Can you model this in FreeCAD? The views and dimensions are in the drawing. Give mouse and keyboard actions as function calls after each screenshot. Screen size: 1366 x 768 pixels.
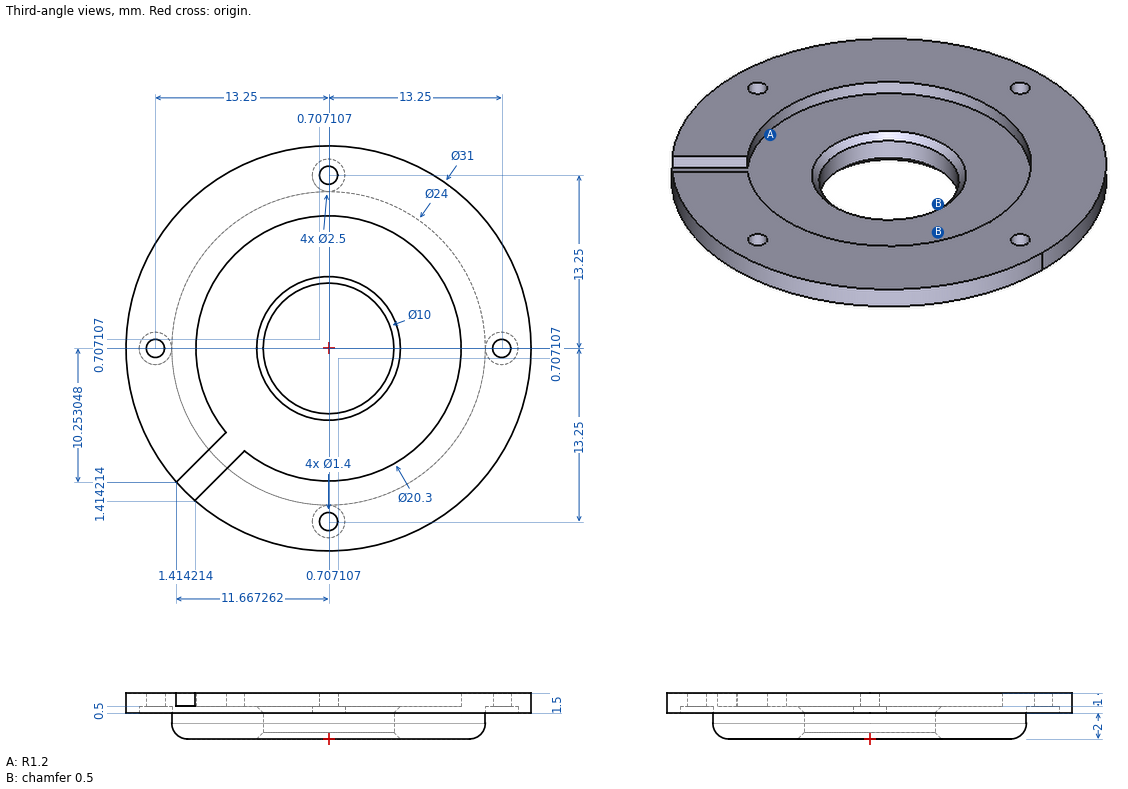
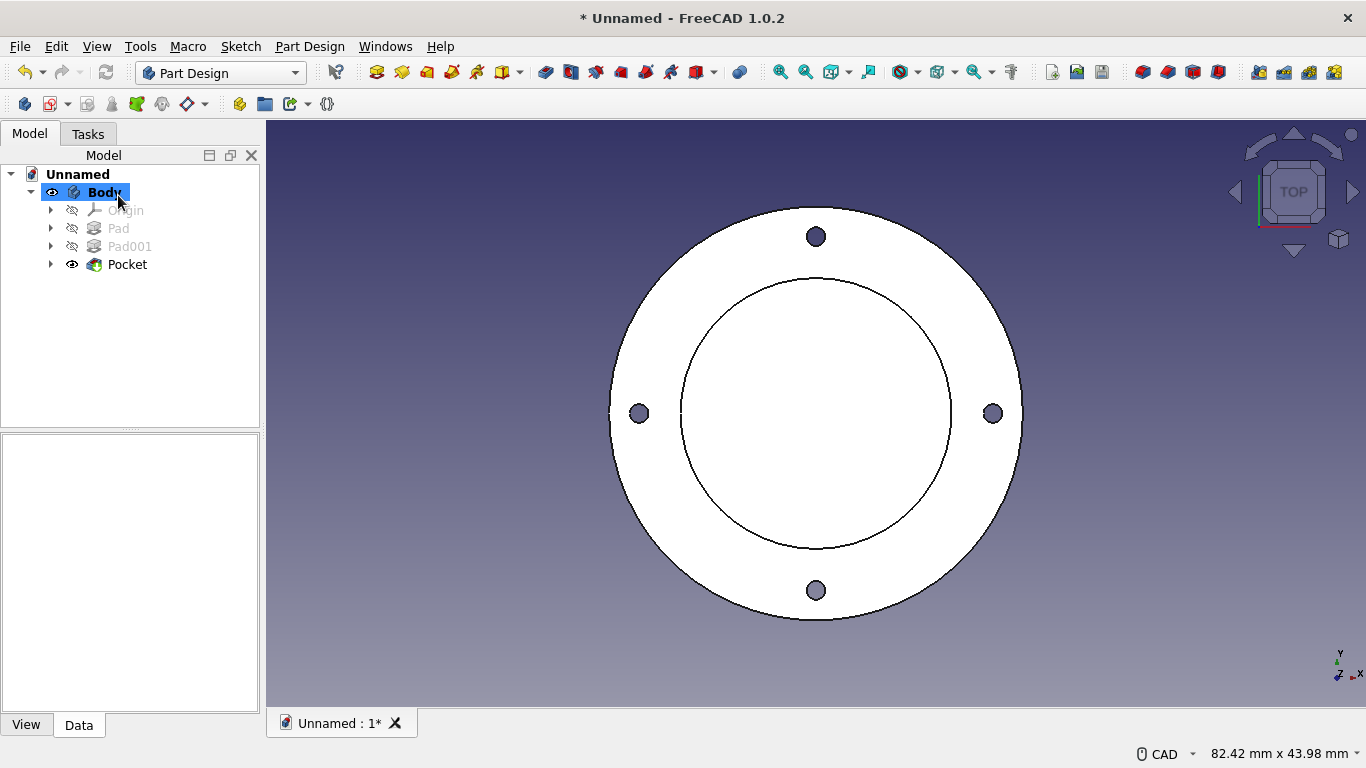
key(1)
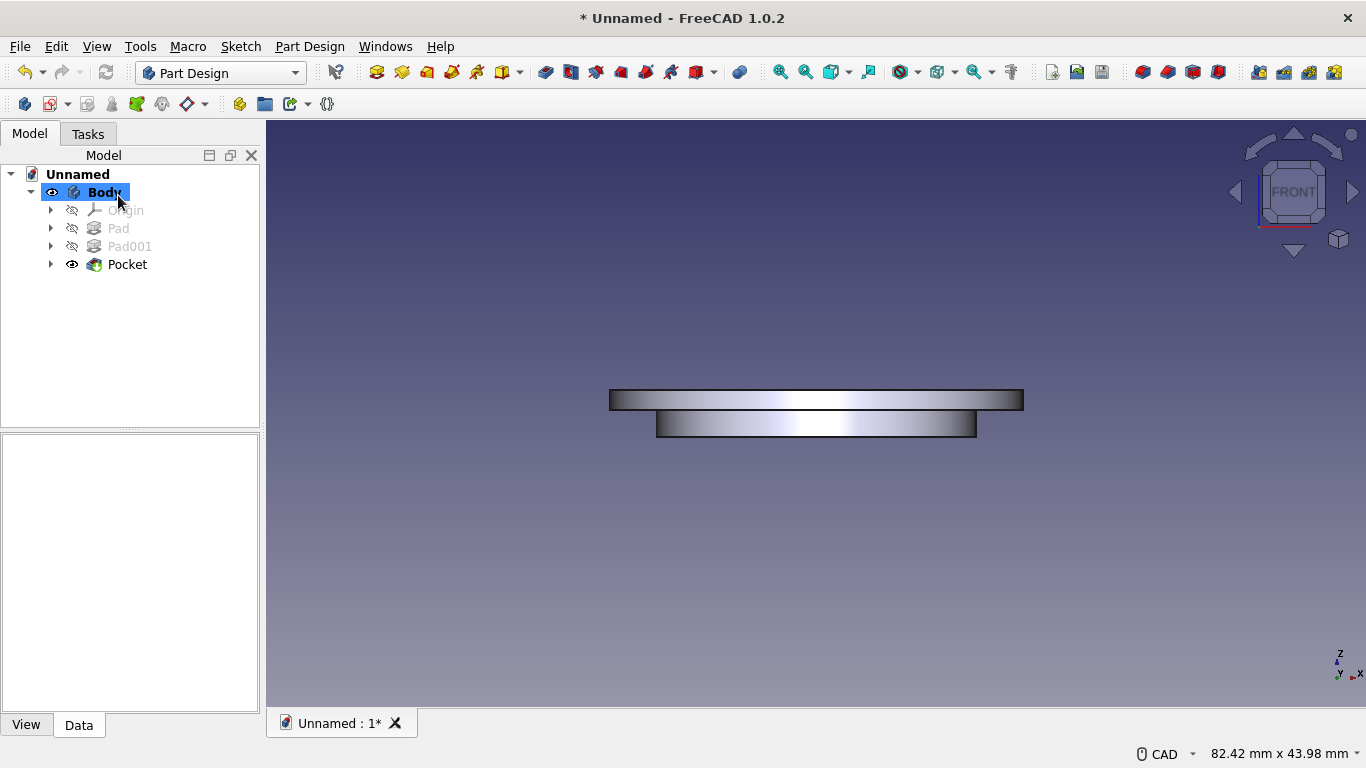
key(v)
key(f)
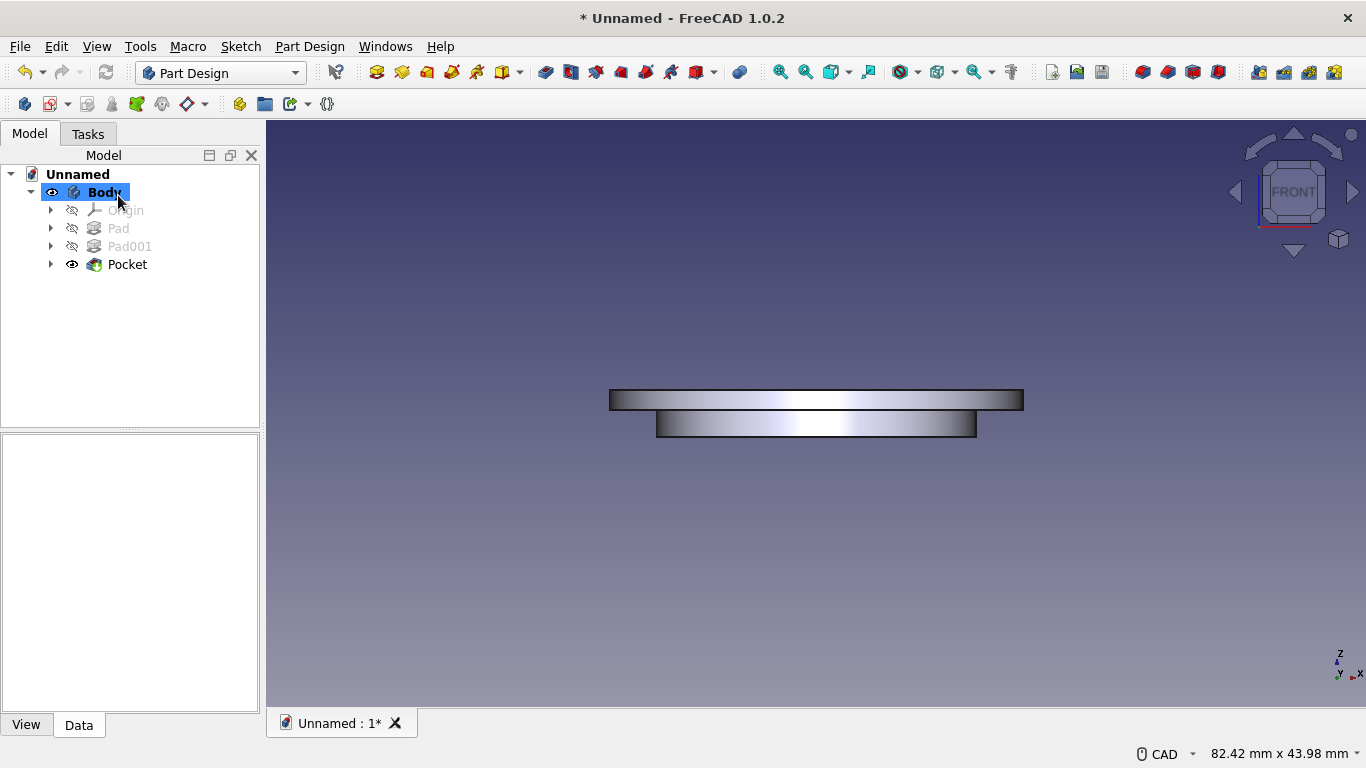
click(686, 436)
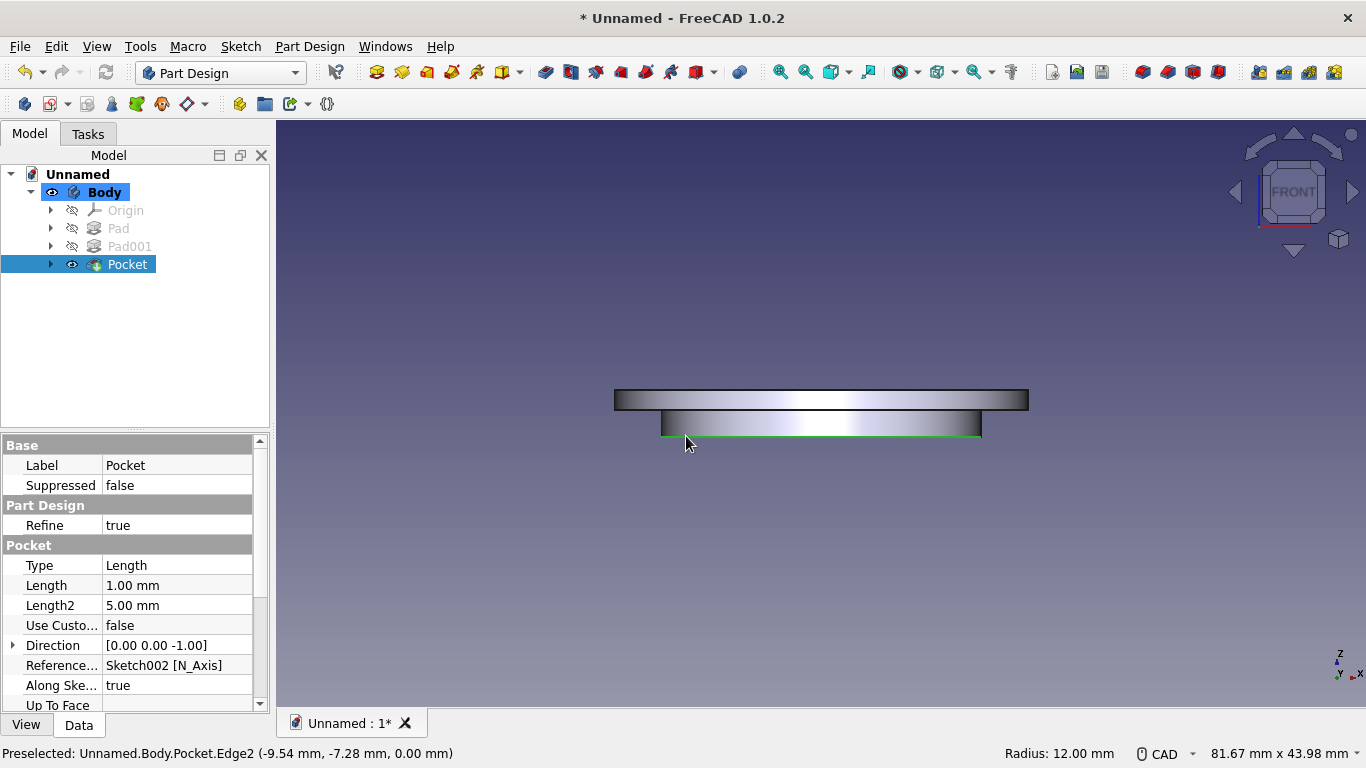
click(1143, 72)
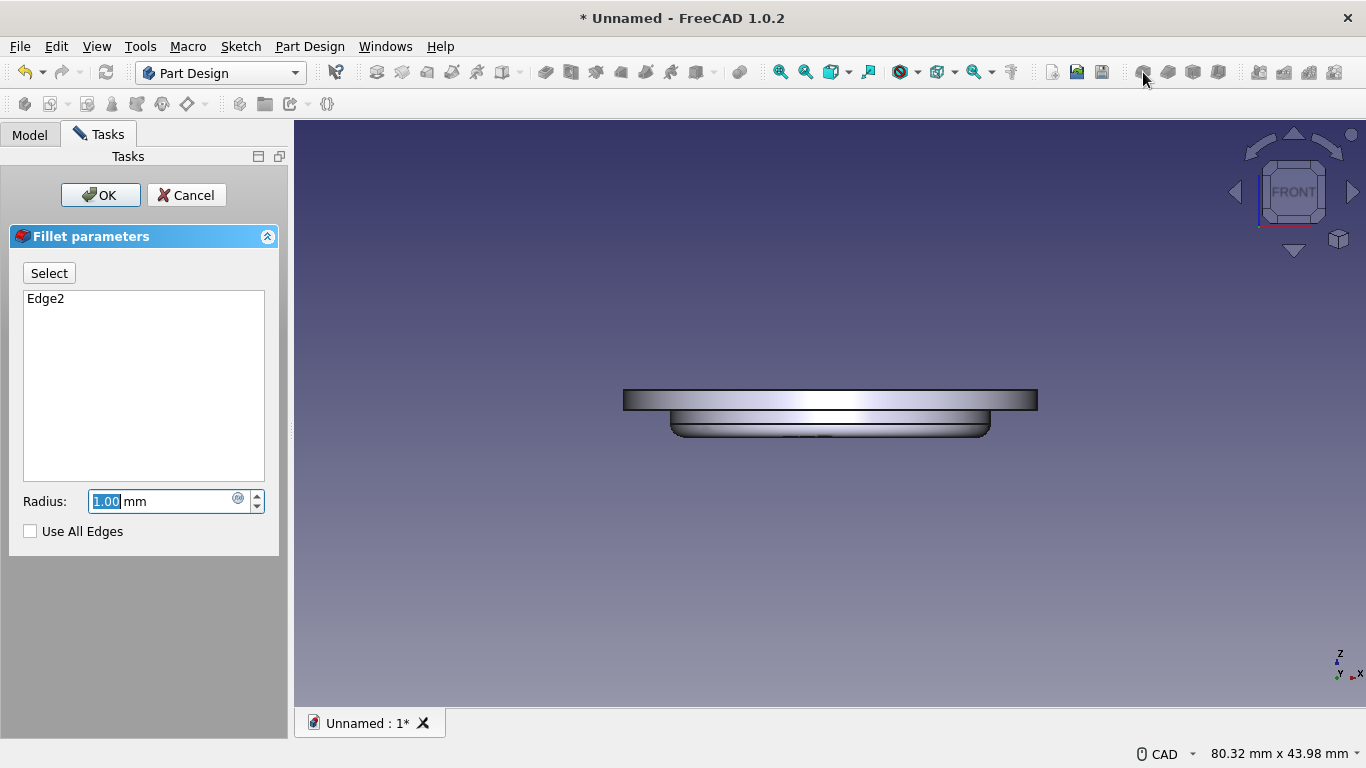
text(1.2)
key(Tab)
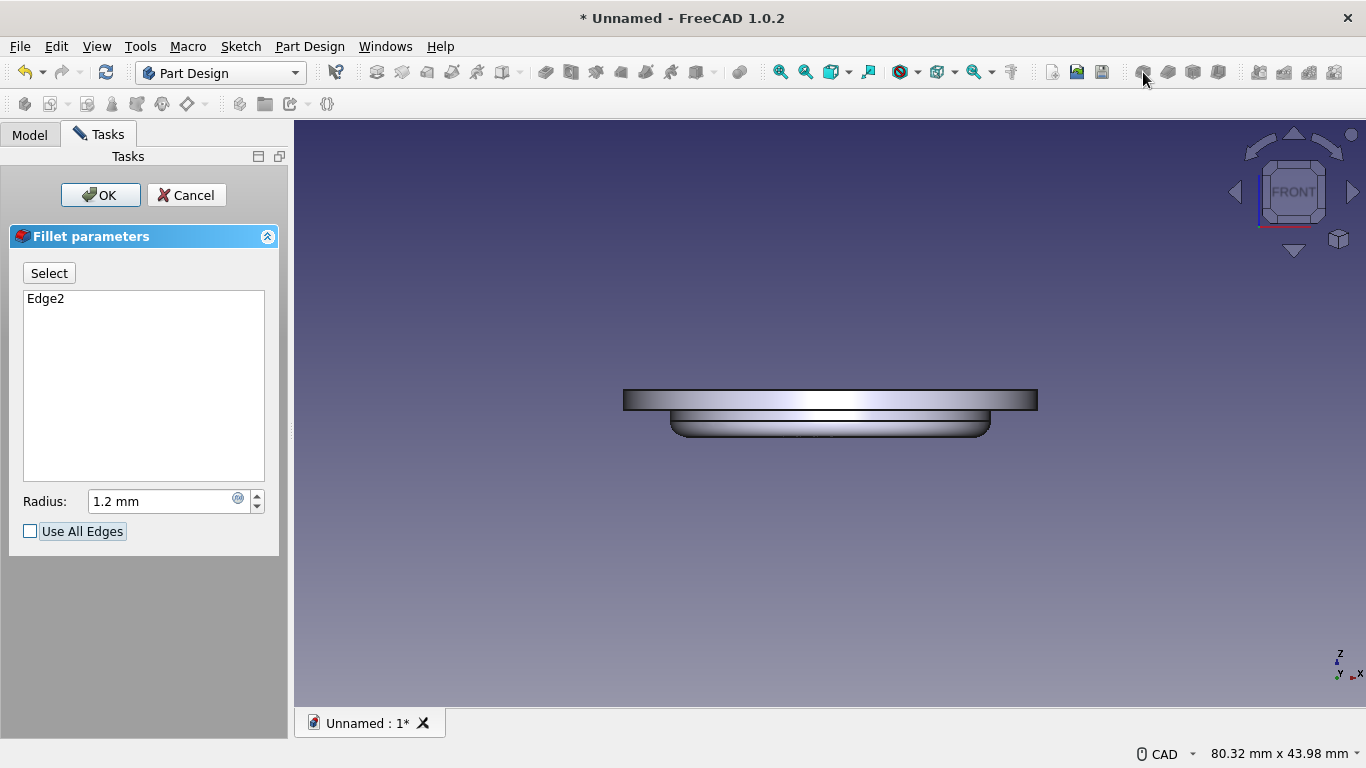
click(101, 195)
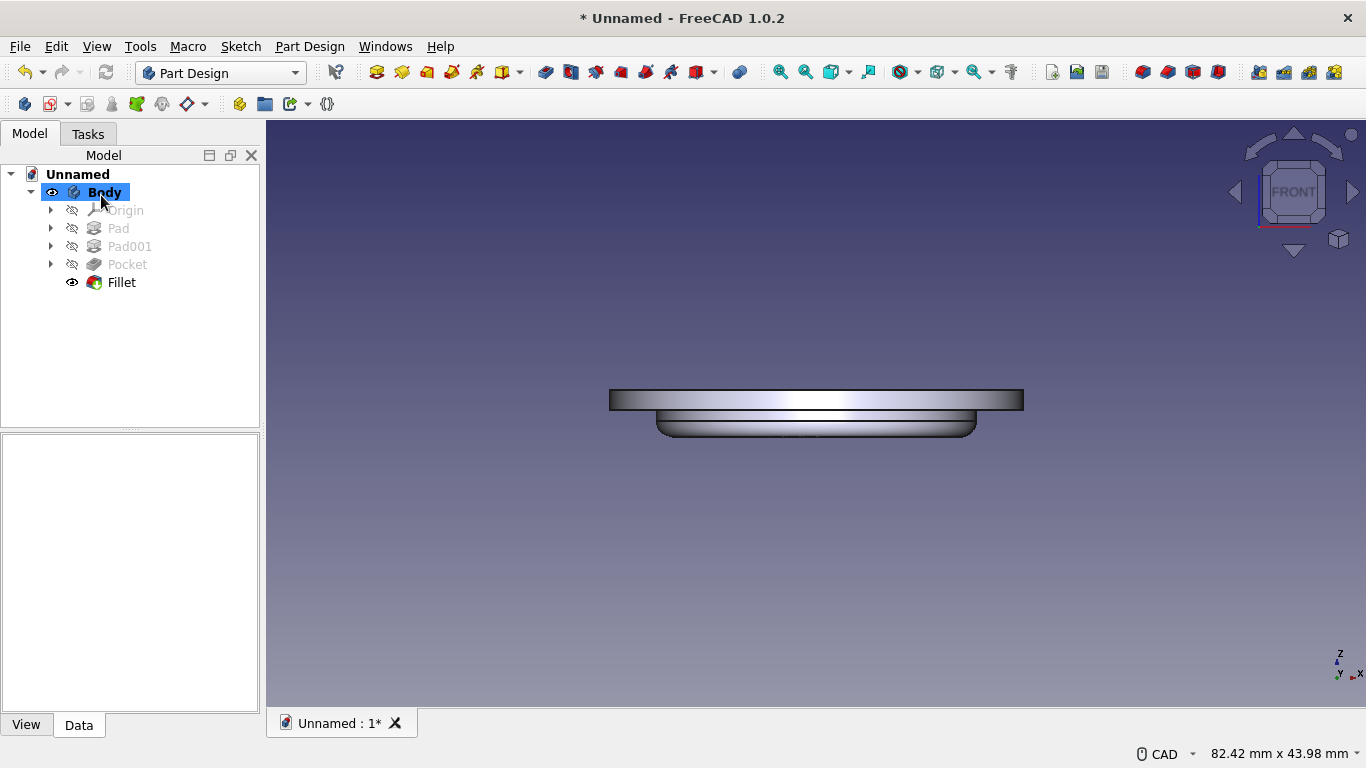
click(781, 72)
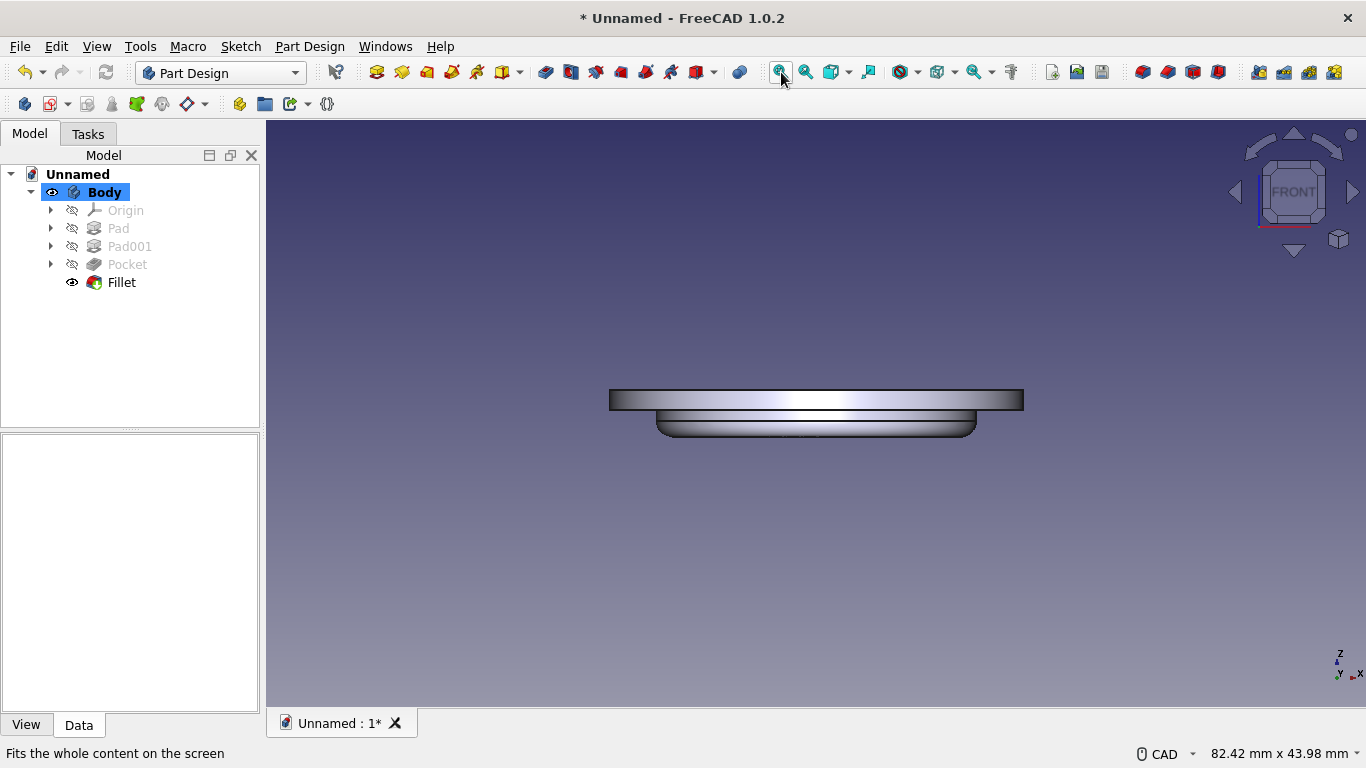
key(5)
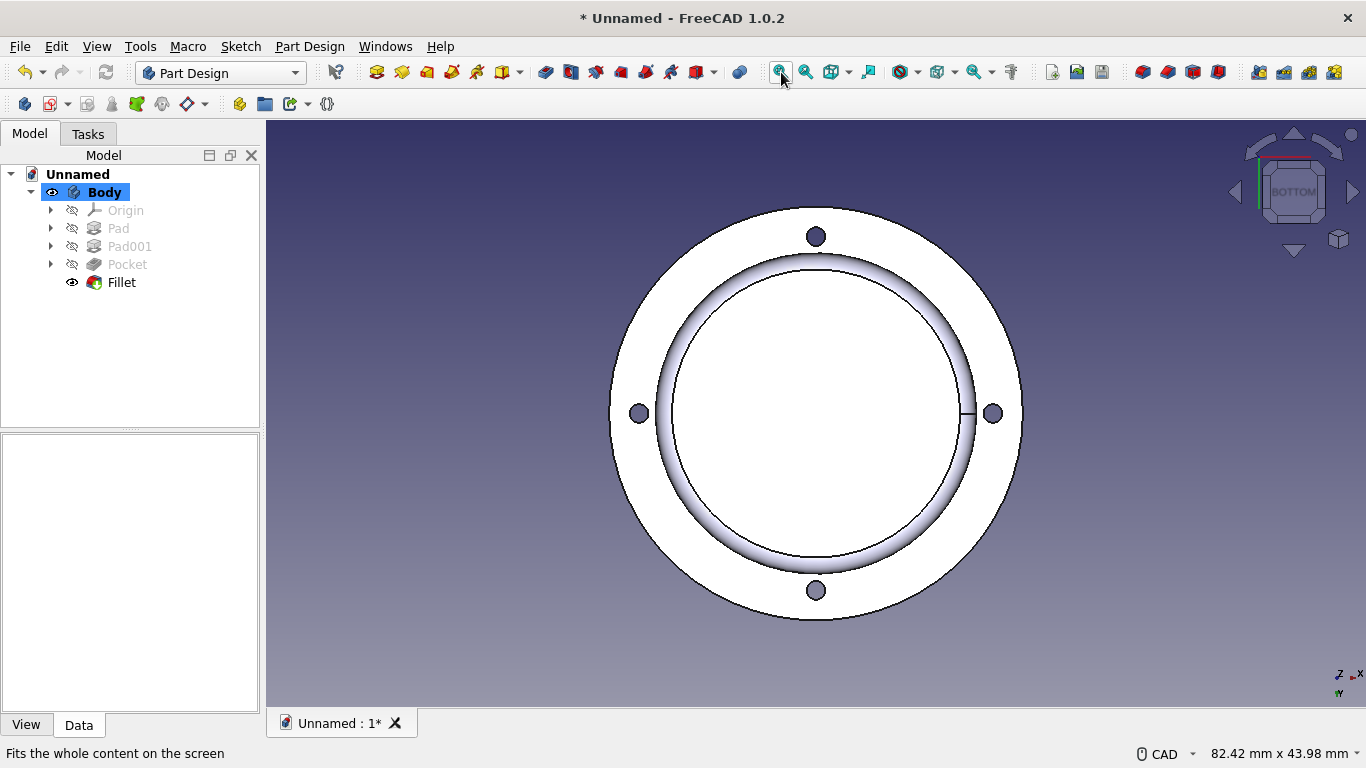
click(875, 235)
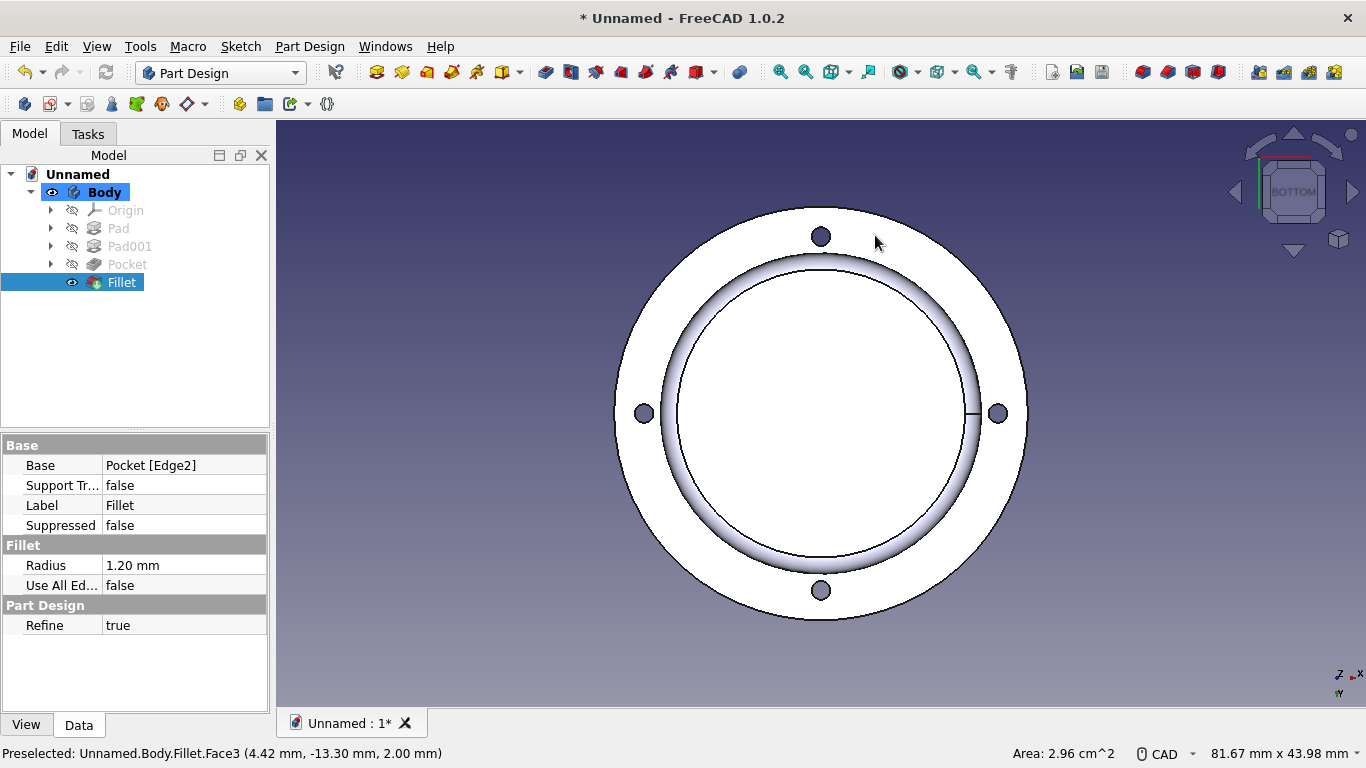
click(50, 104)